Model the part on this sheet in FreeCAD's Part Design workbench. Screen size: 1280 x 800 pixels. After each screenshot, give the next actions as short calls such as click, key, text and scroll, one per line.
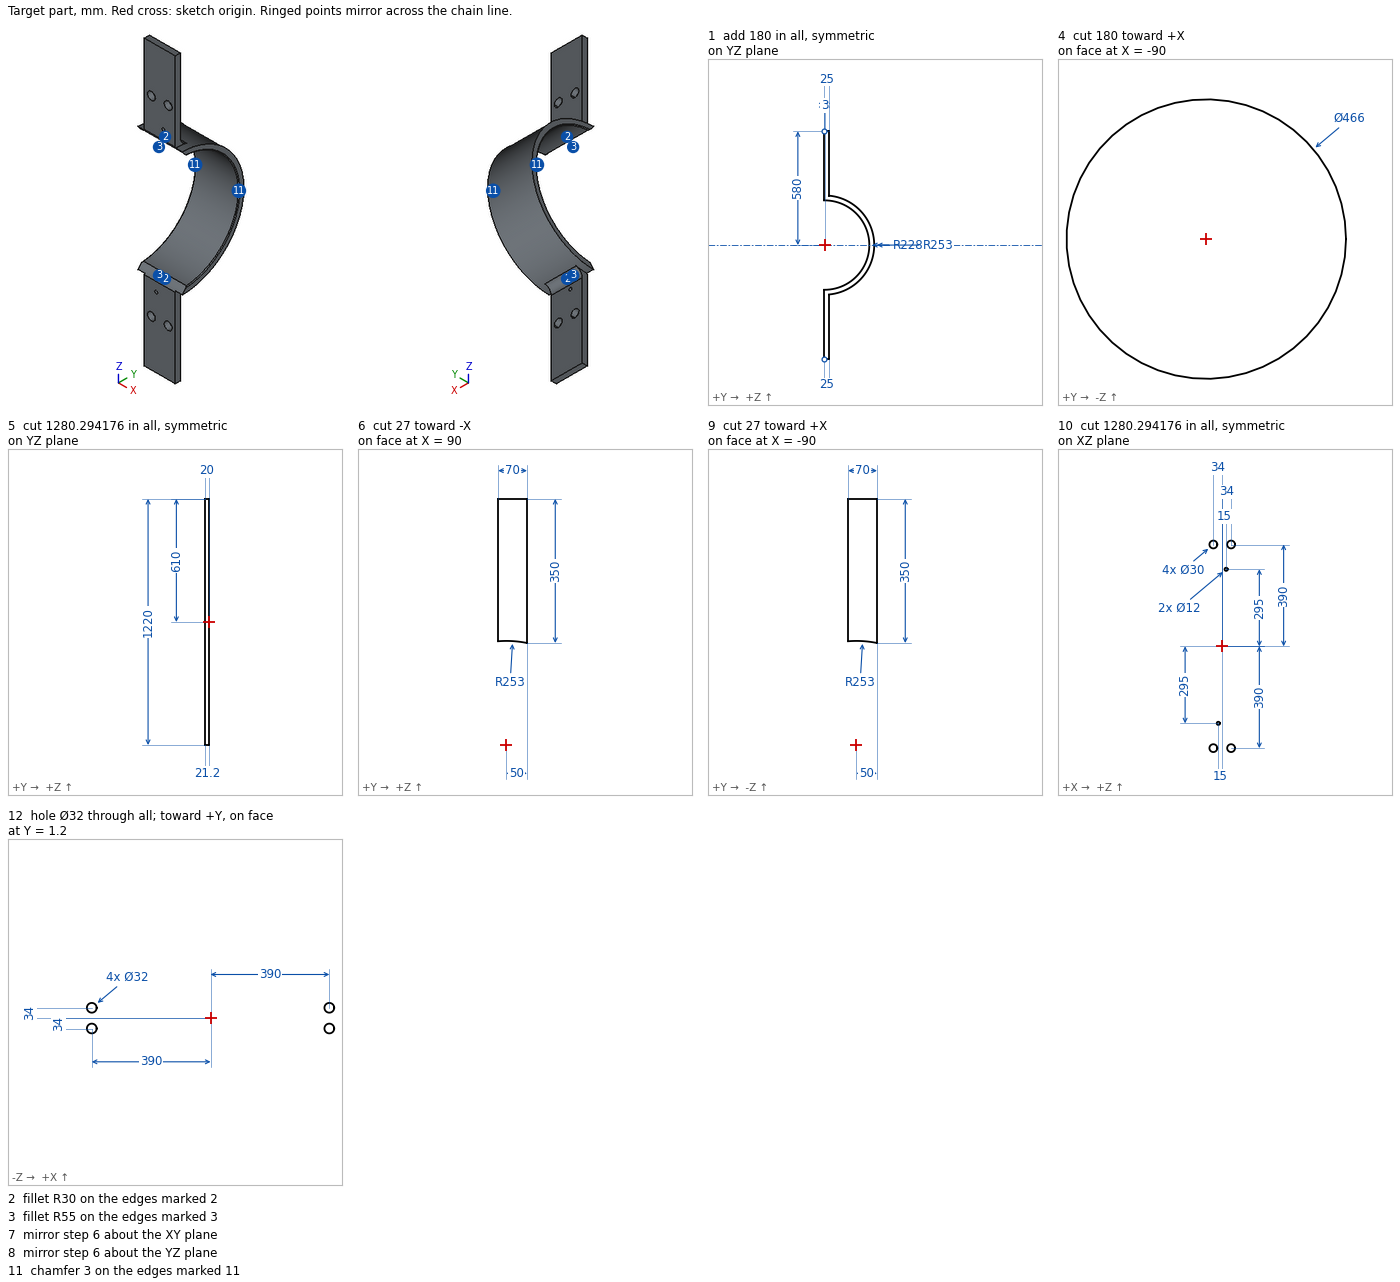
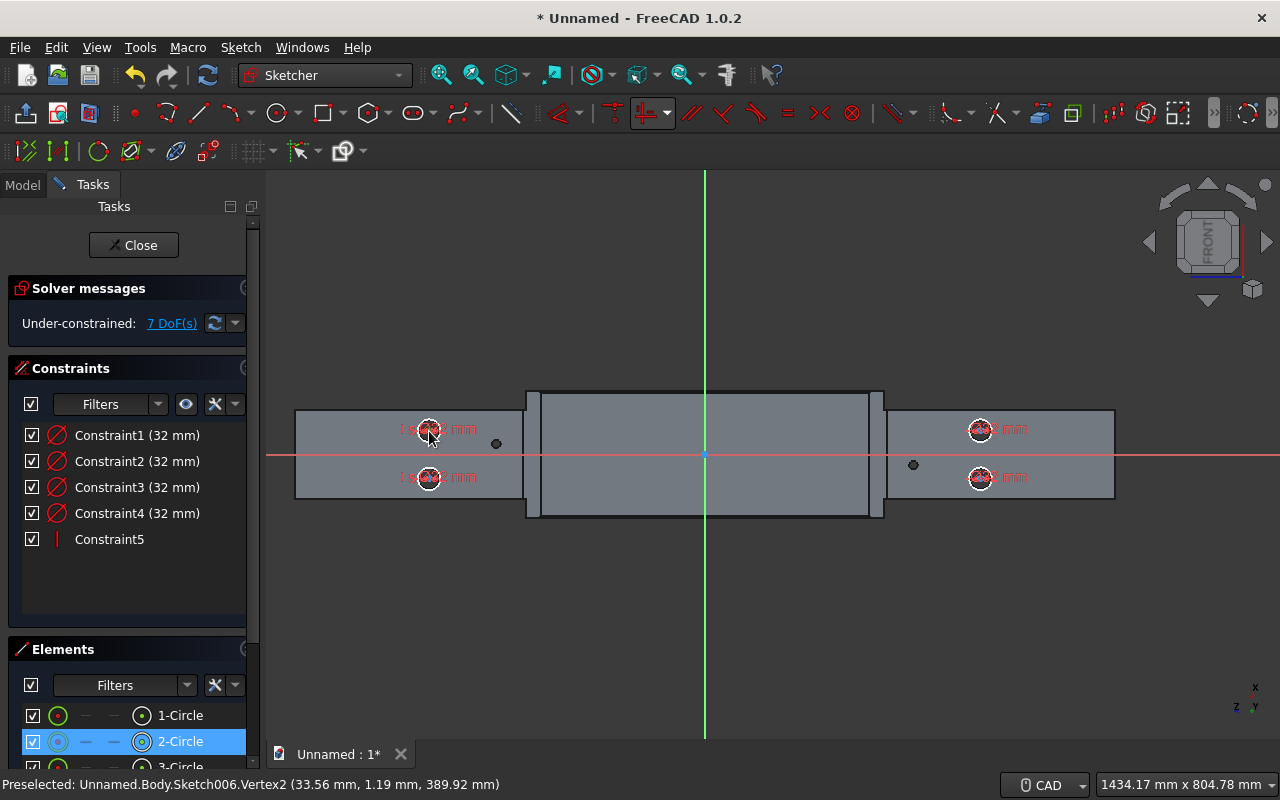
click(980, 431)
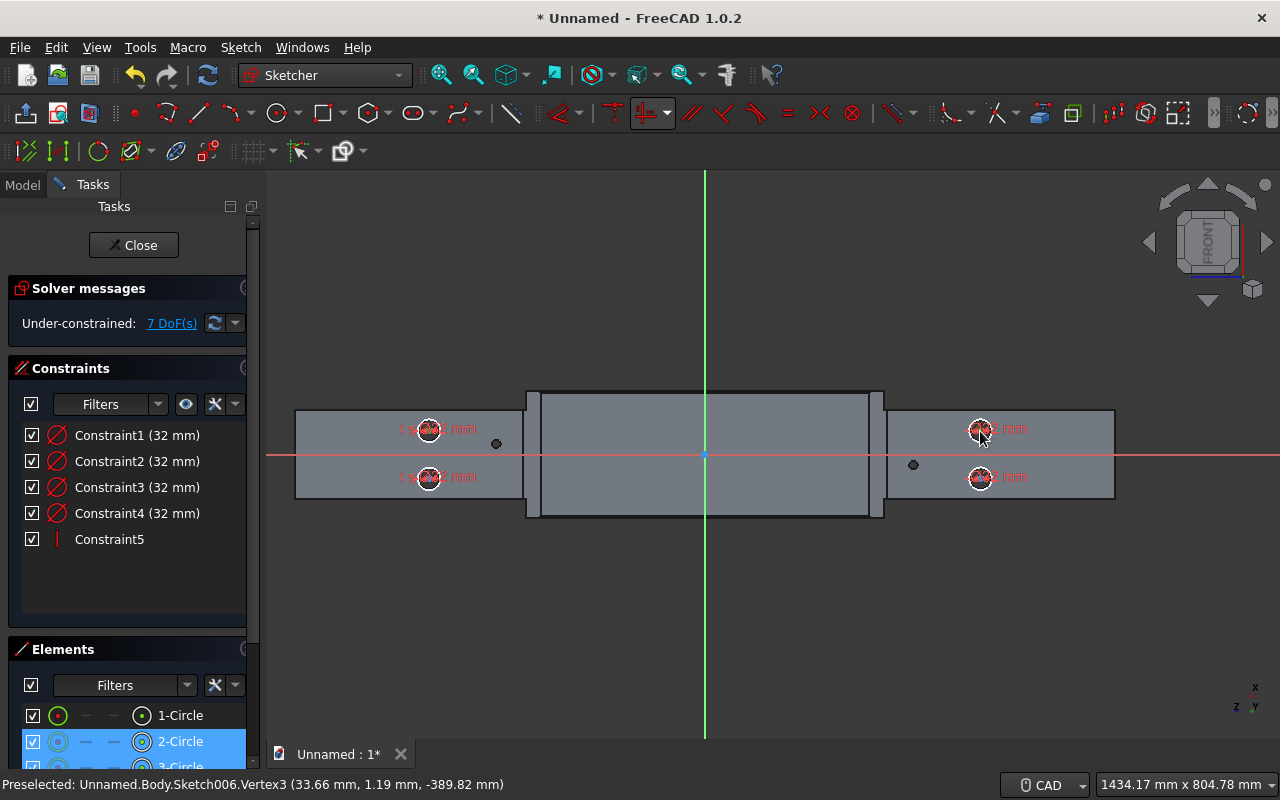
key(h)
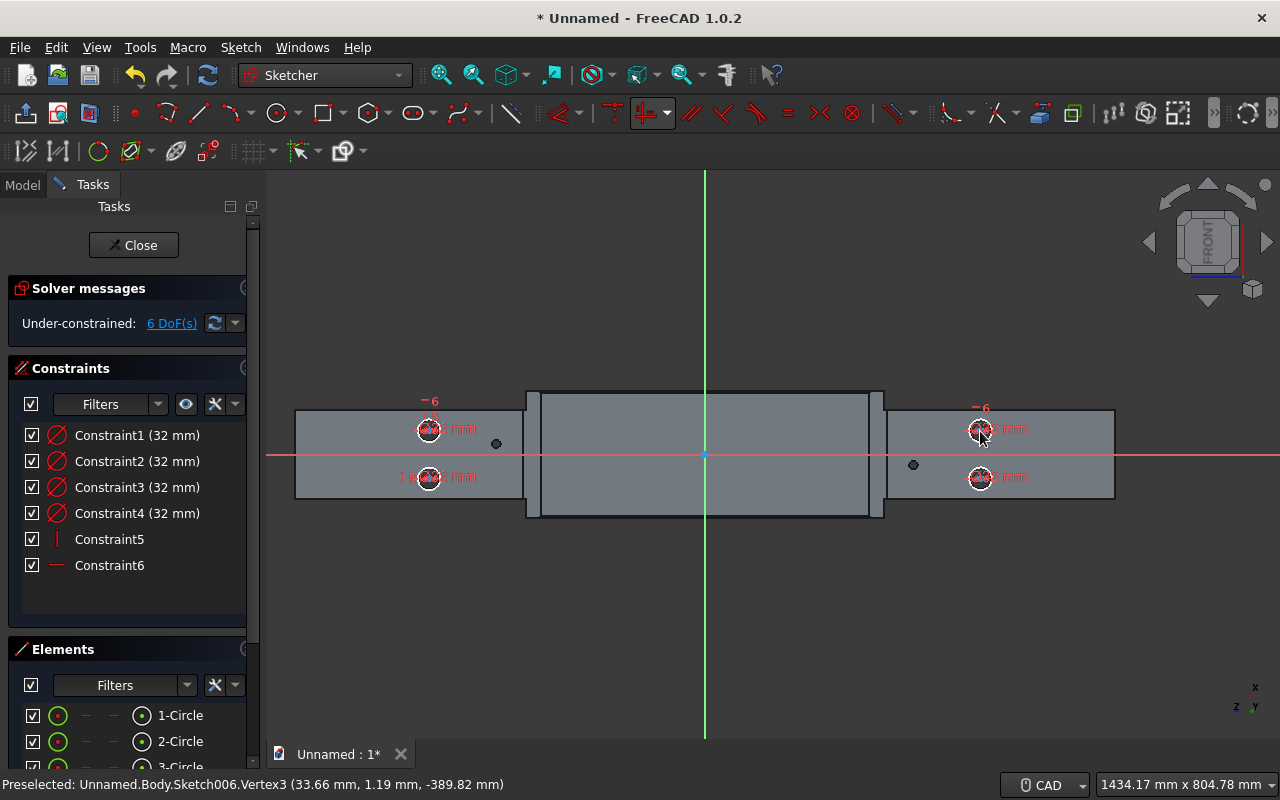
click(980, 431)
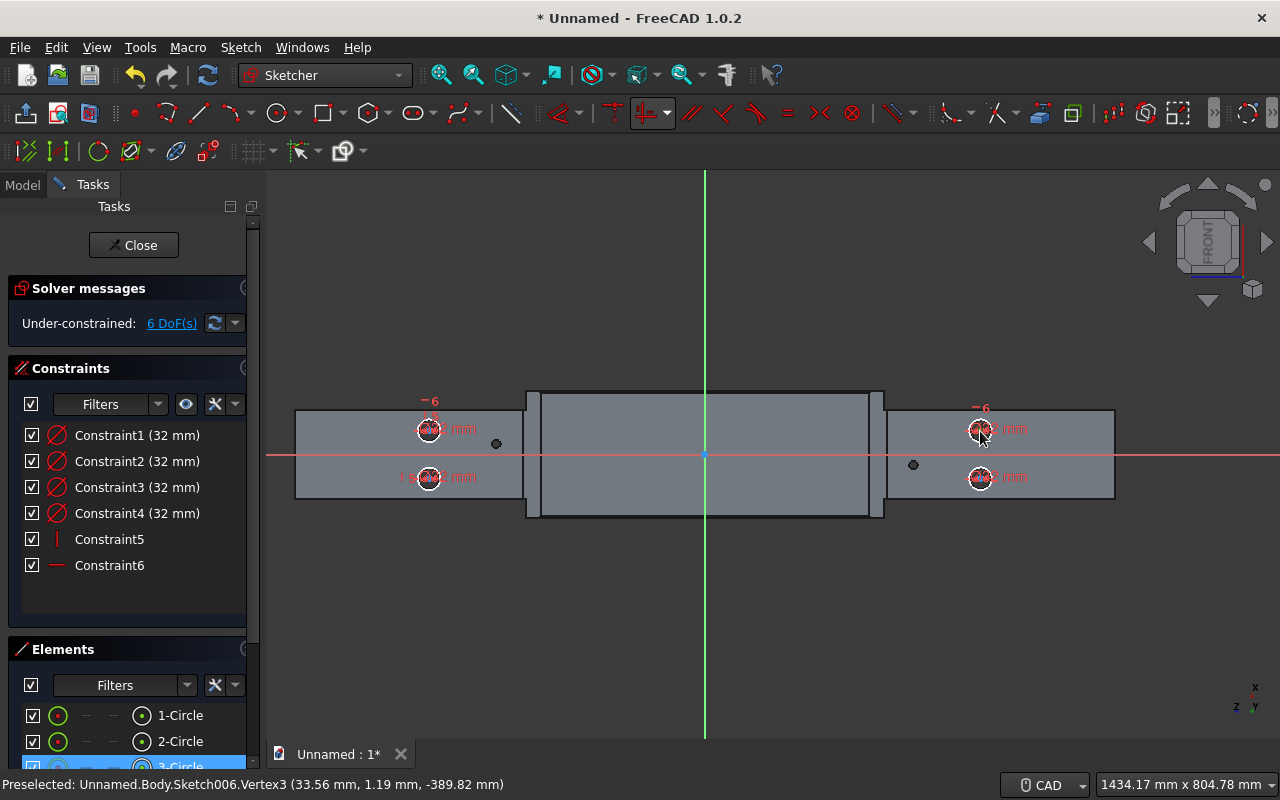
click(980, 479)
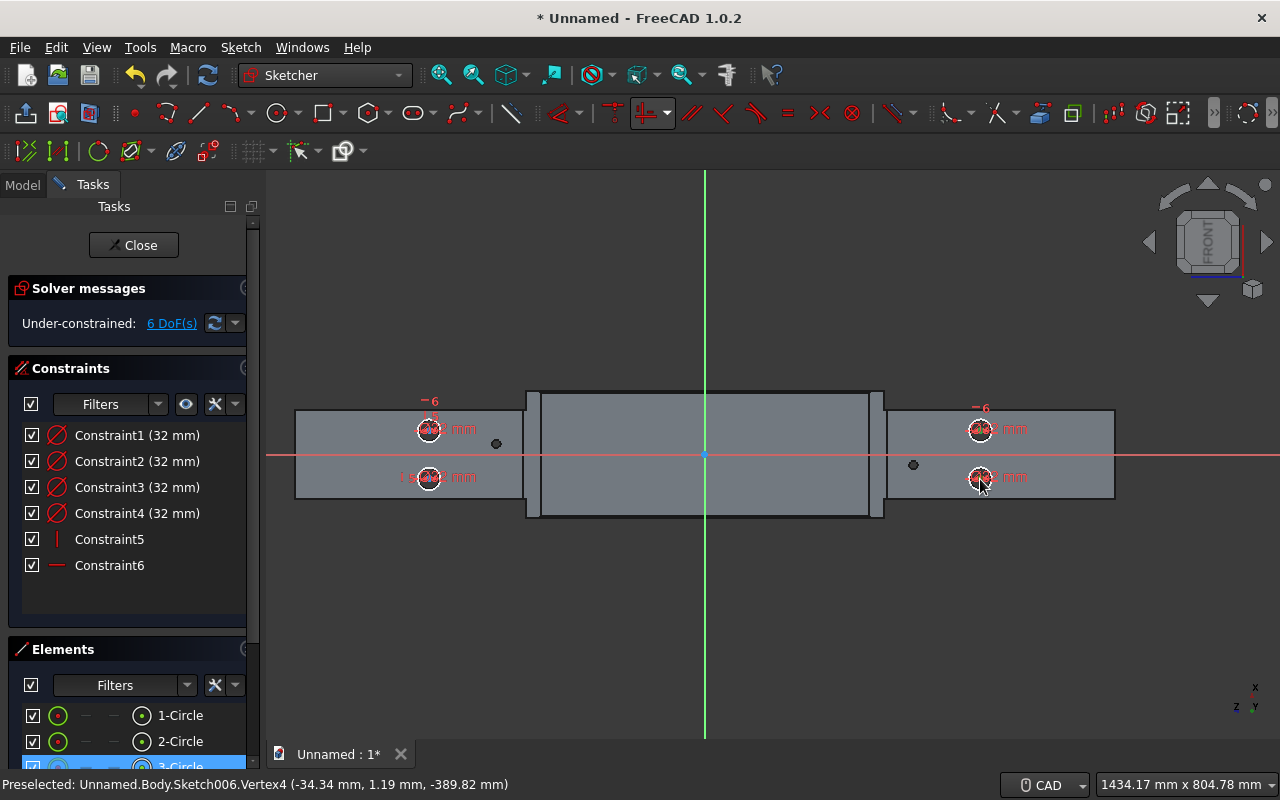
key(v)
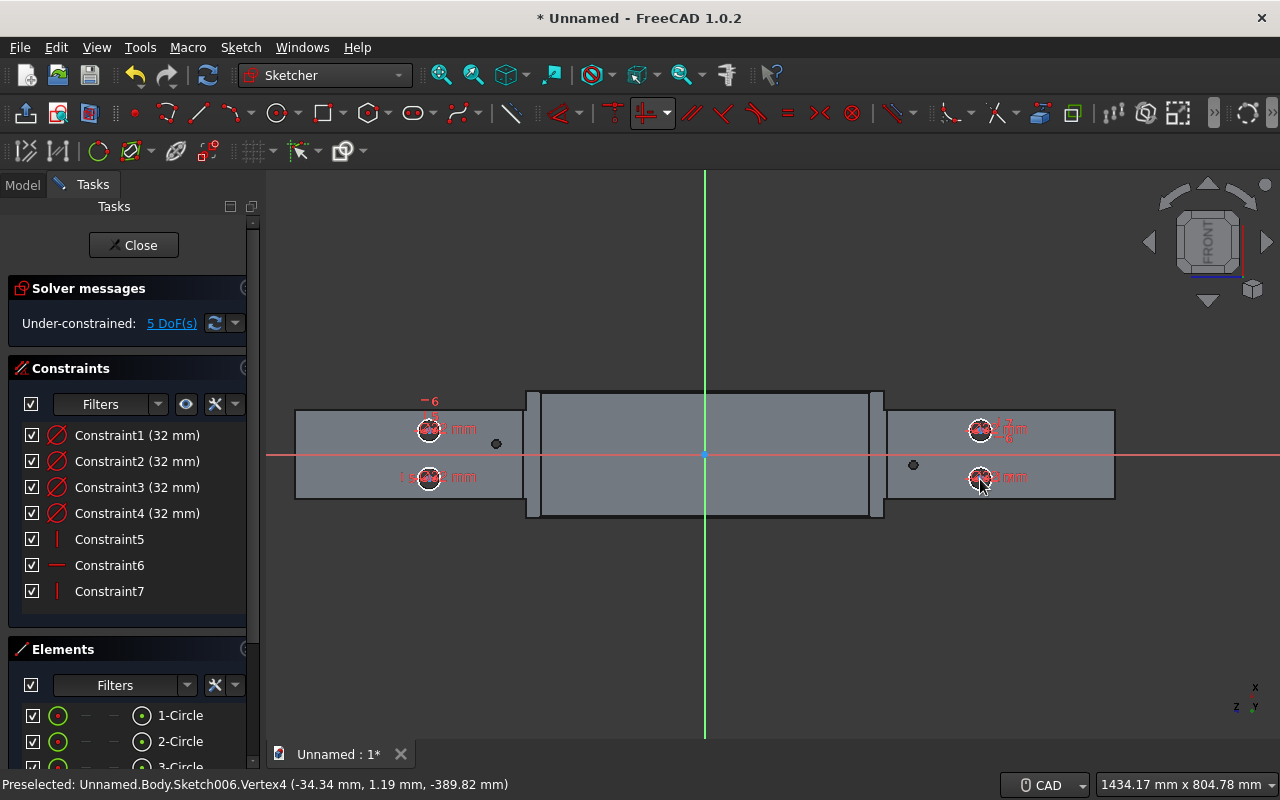
click(429, 479)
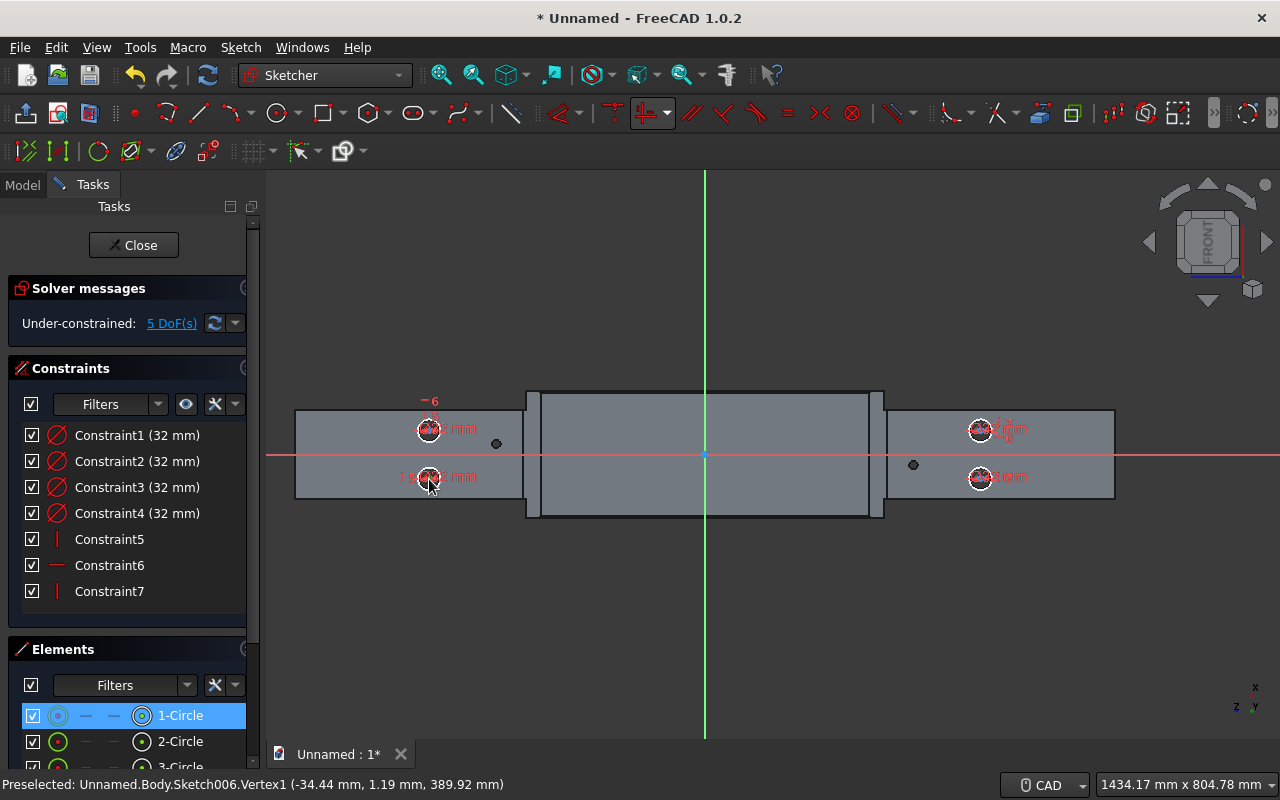
click(980, 479)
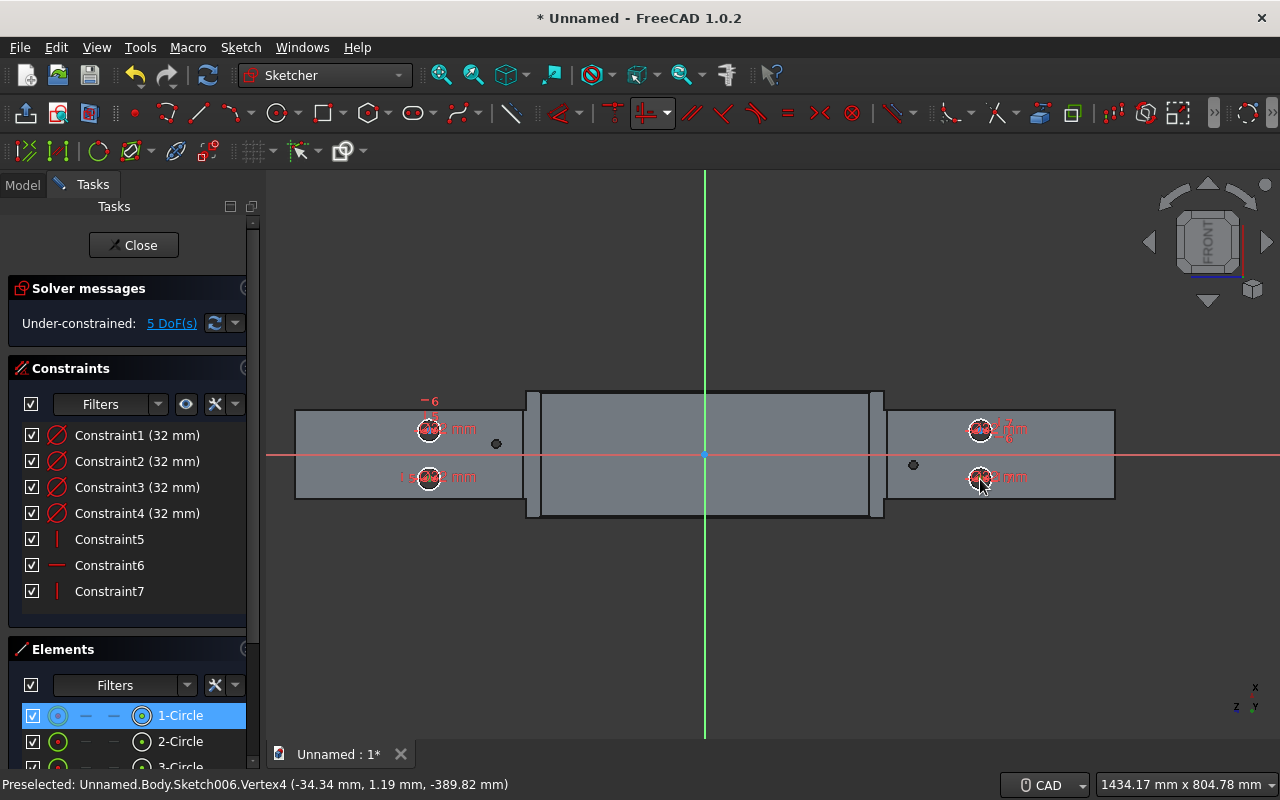
click(670, 114)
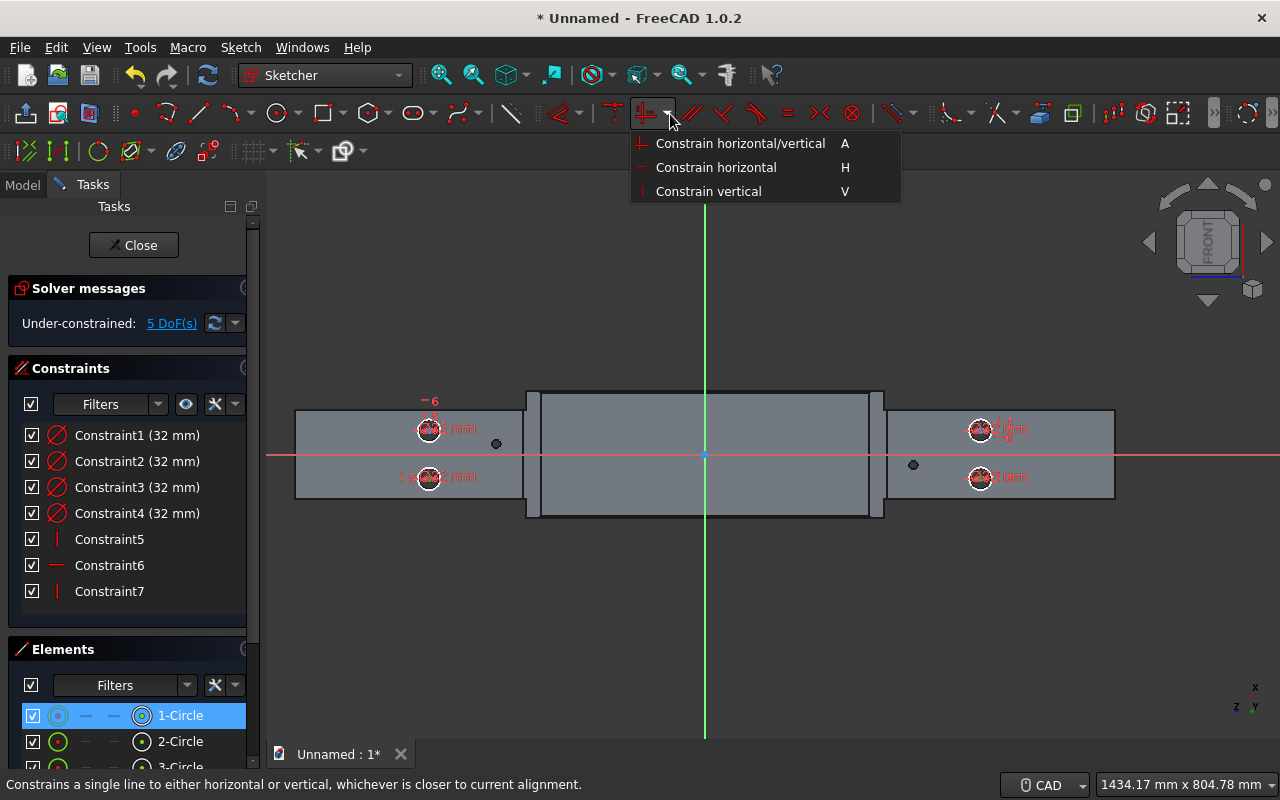
click(766, 167)